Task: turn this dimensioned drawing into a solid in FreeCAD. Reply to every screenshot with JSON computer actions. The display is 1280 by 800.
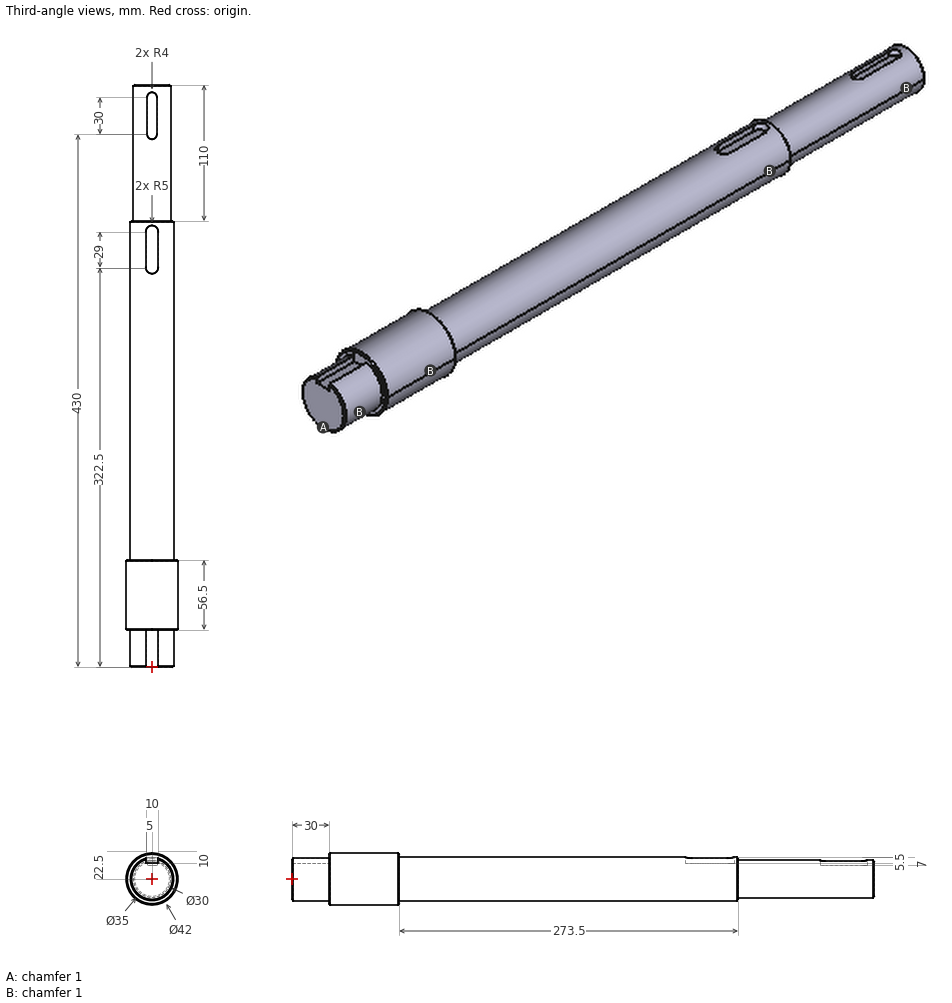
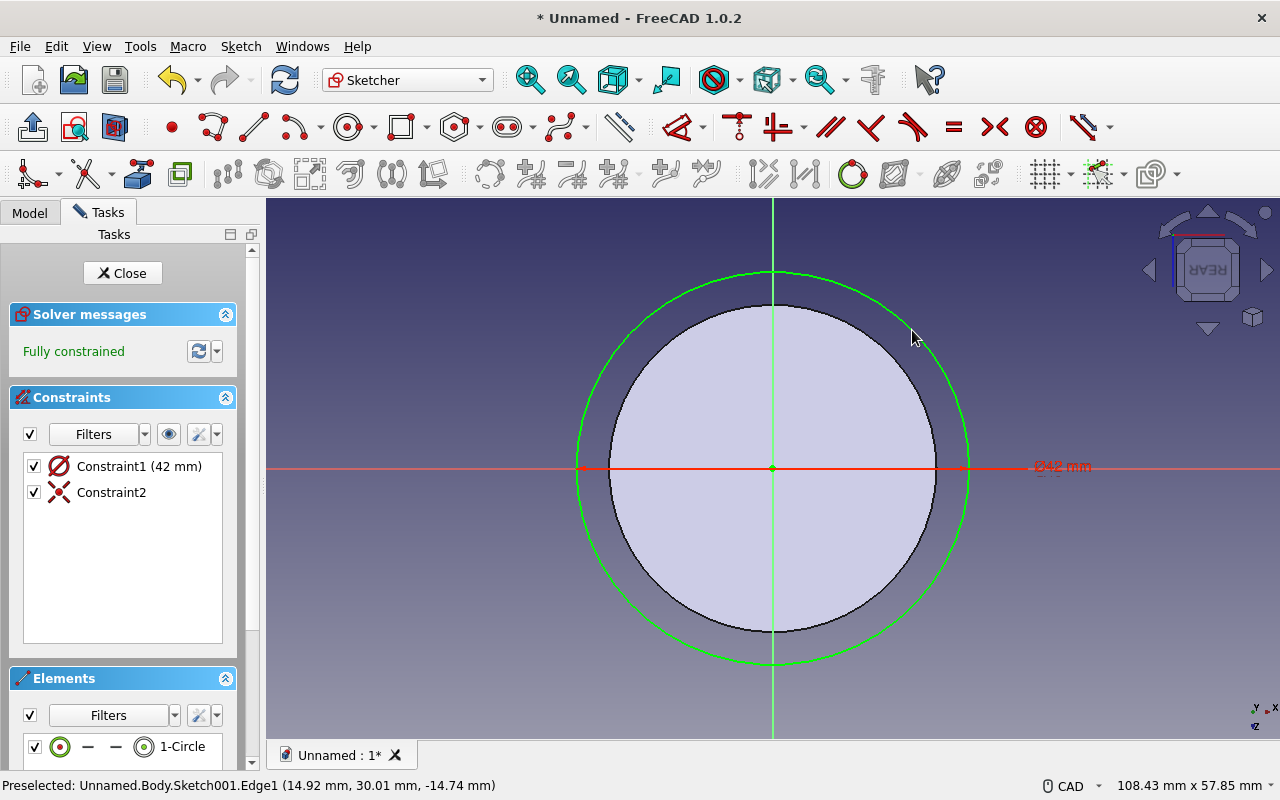
{"action": "left_click", "coordinate": [123, 273]}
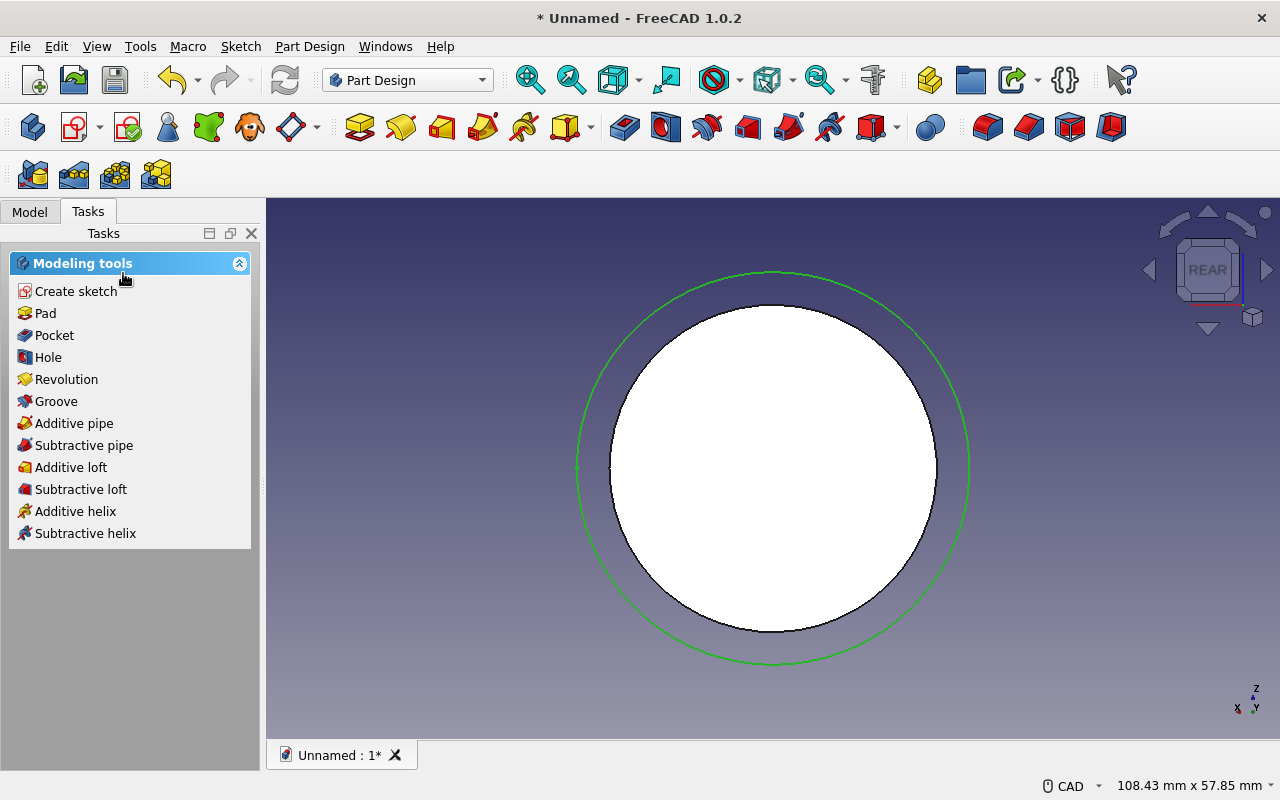
{"action": "left_click", "coordinate": [360, 128]}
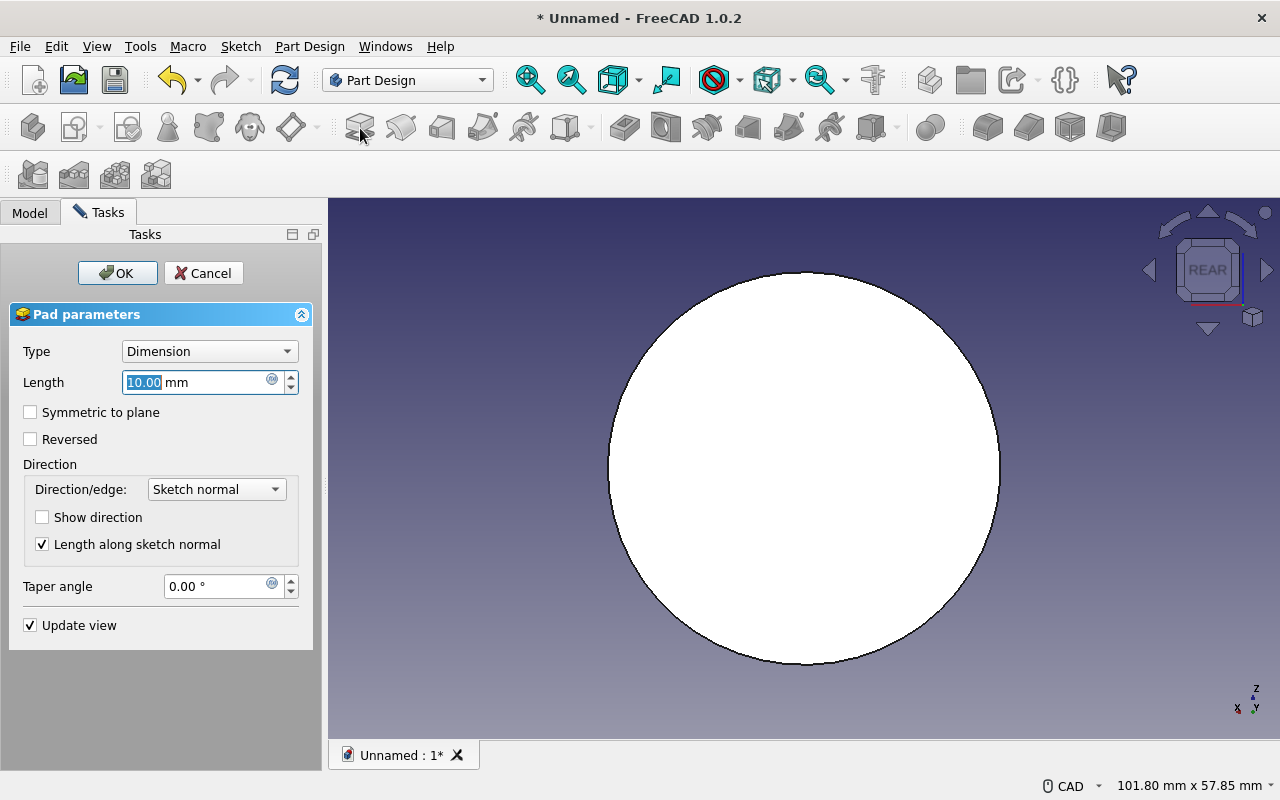
{"action": "type", "text": "56.5"}
{"action": "key", "text": "Tab"}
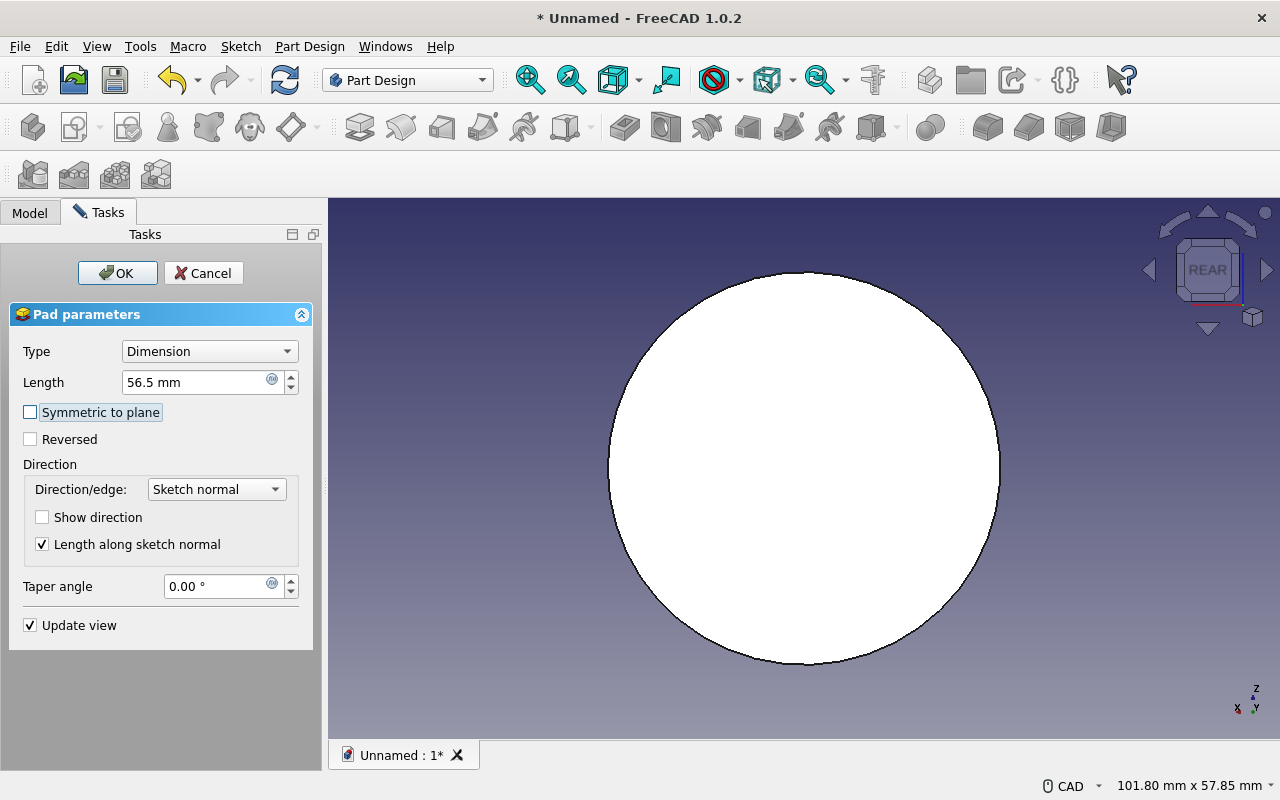
{"action": "left_click", "coordinate": [118, 273]}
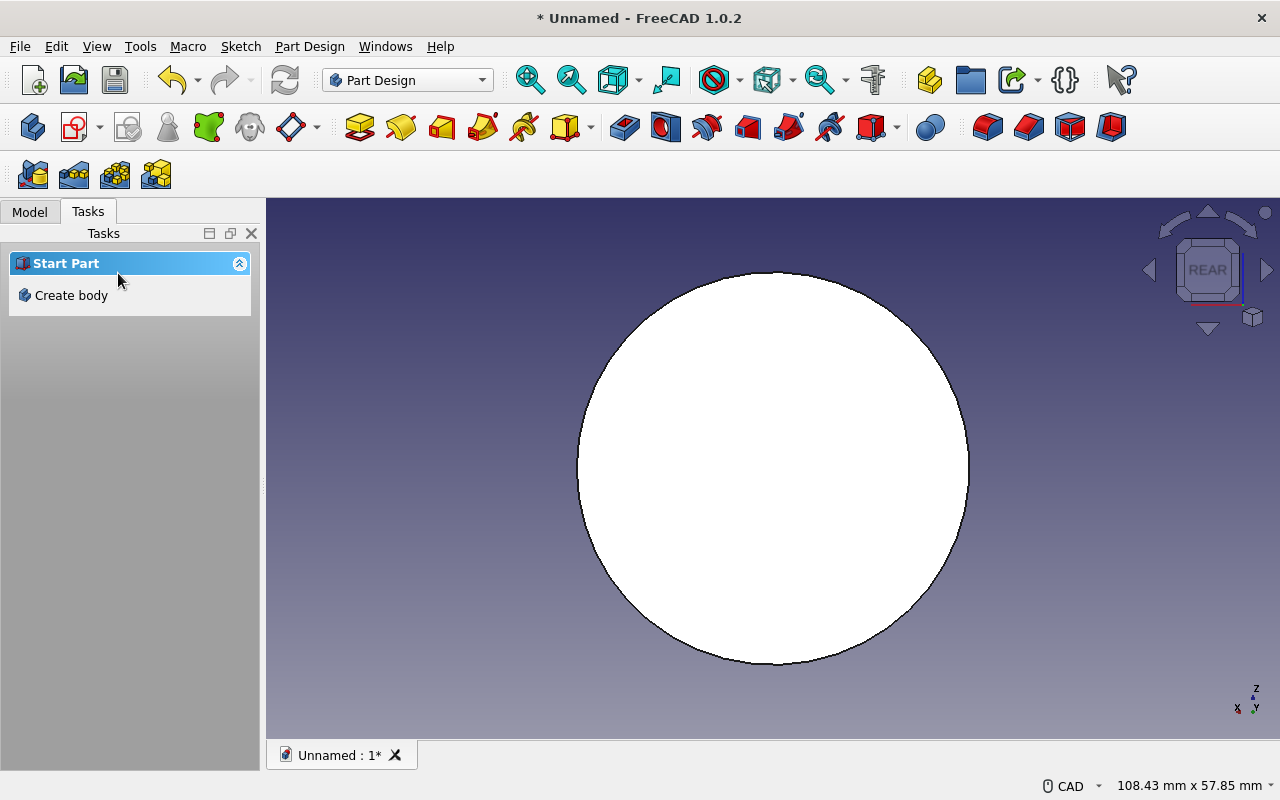
{"action": "left_click", "coordinate": [773, 468]}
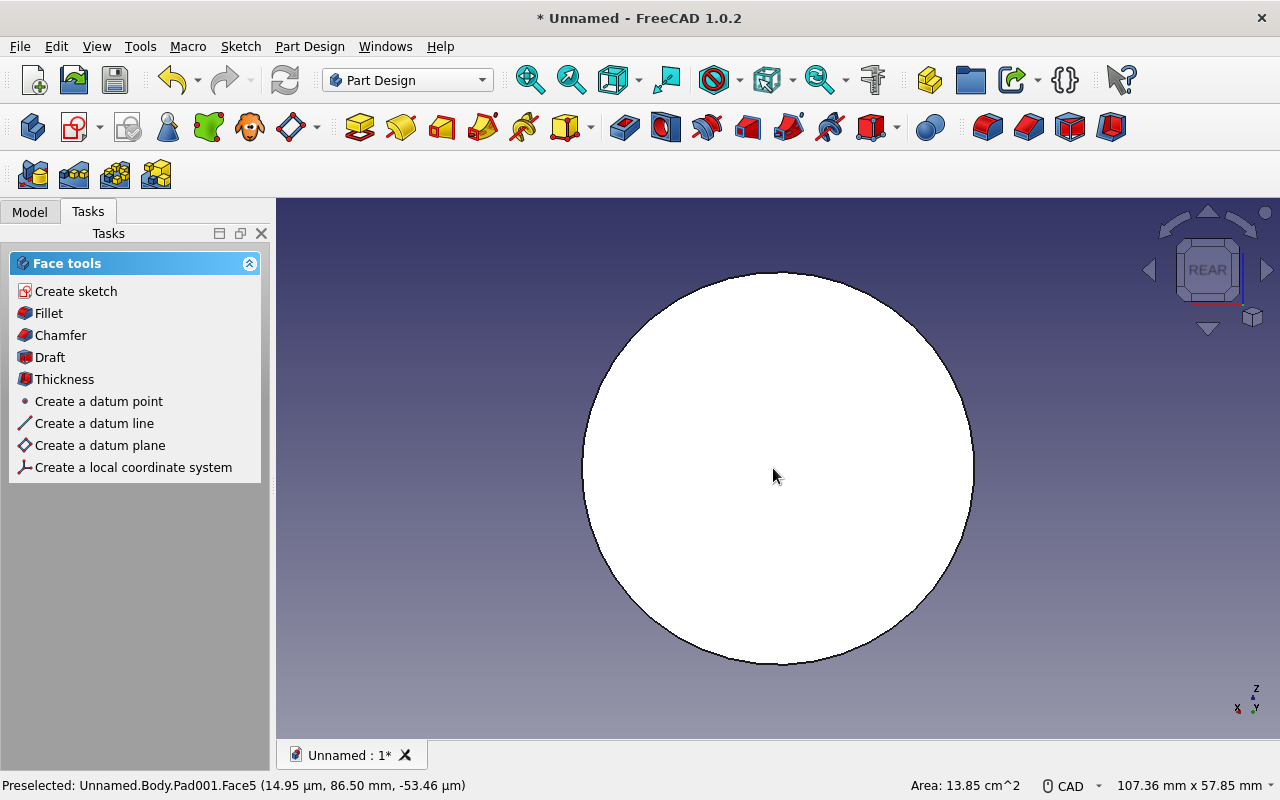
{"action": "left_click", "coordinate": [74, 128]}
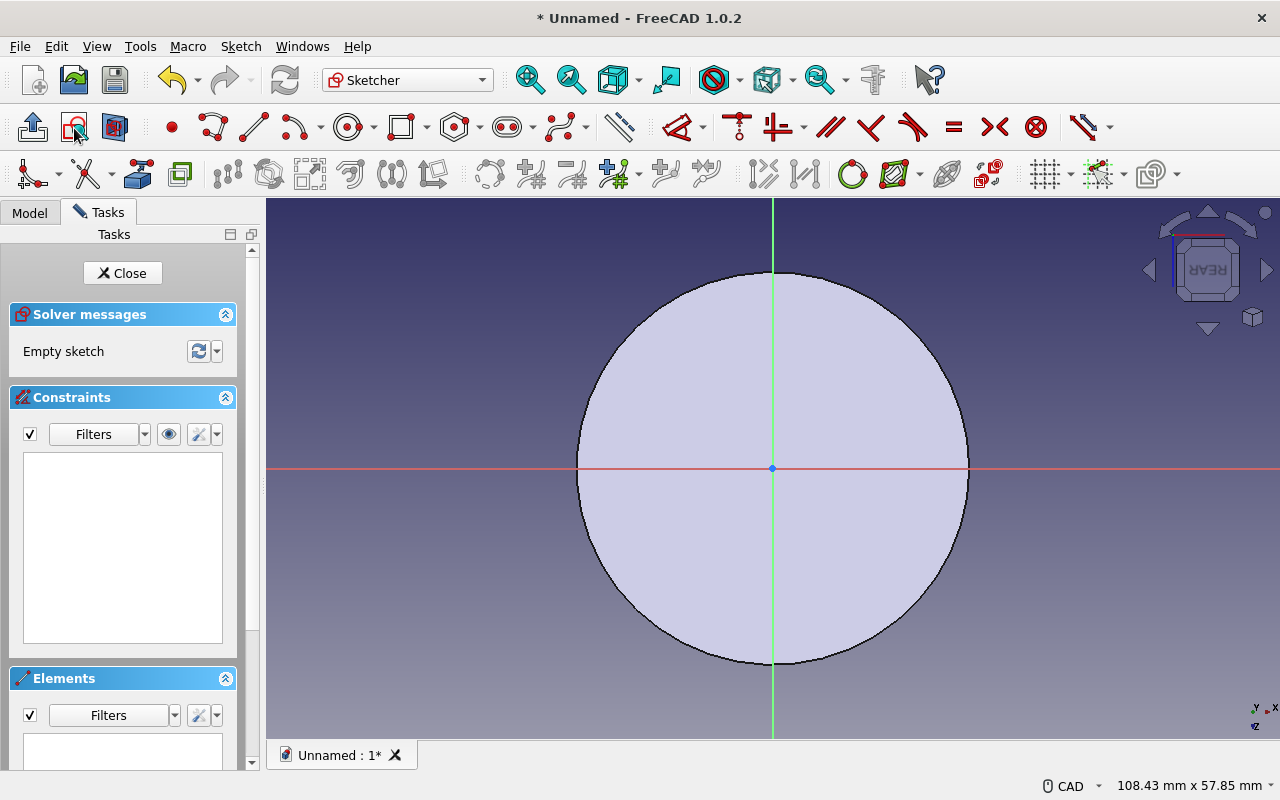
{"action": "left_click", "coordinate": [348, 128]}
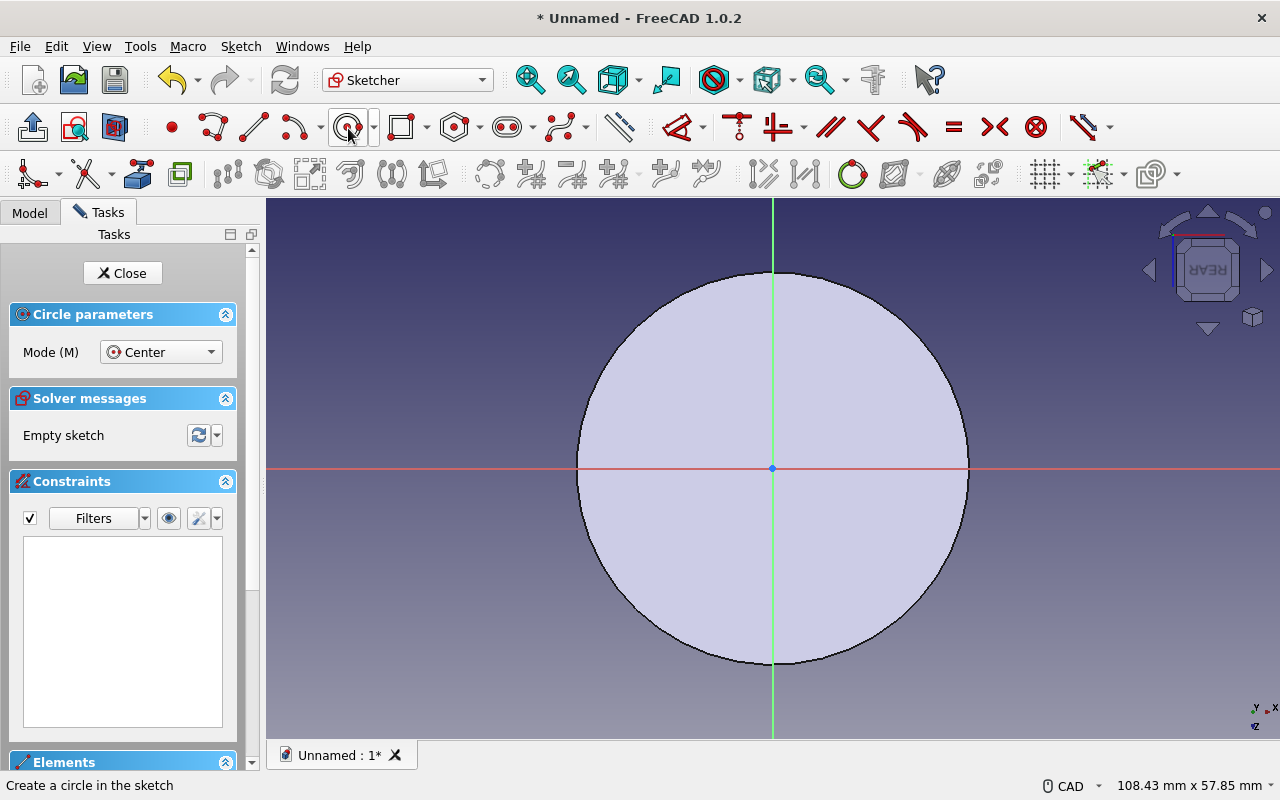
{"action": "left_click", "coordinate": [773, 468]}
{"action": "mouse_move", "coordinate": [889, 353]}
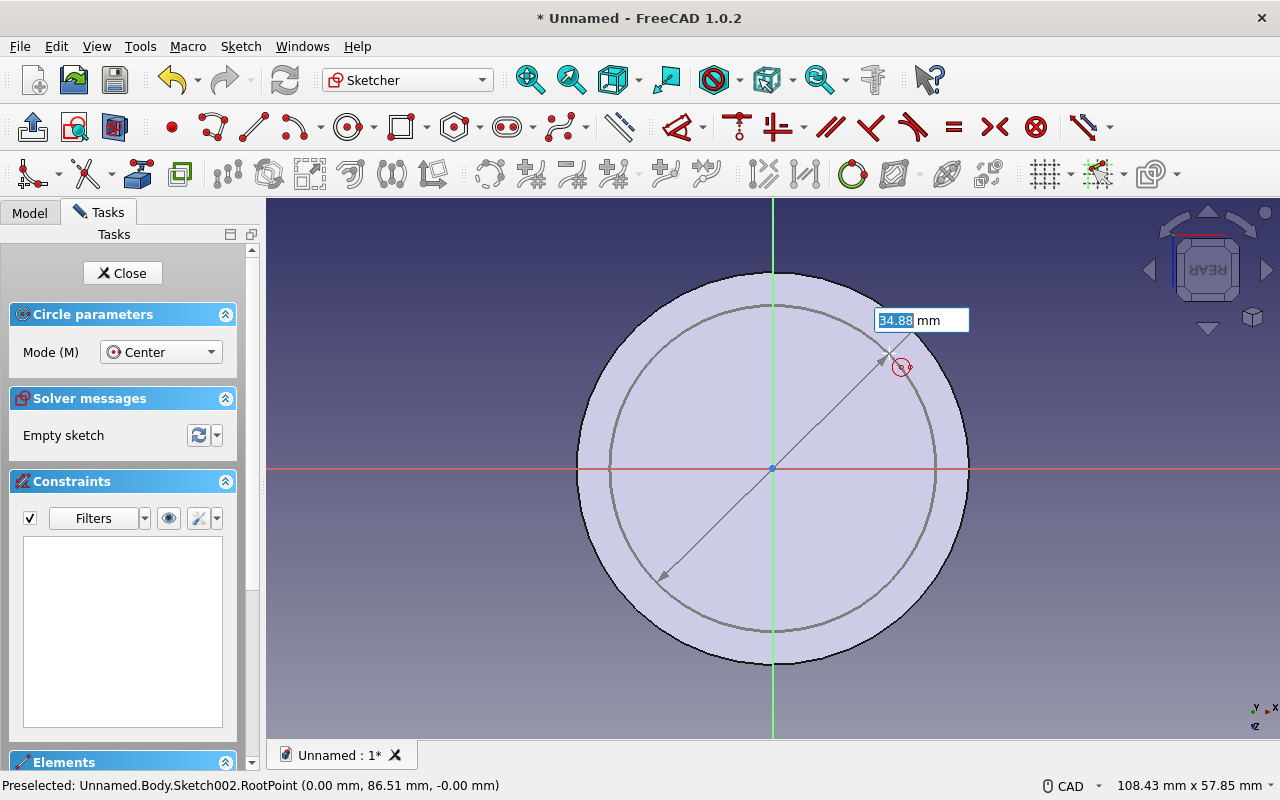
{"action": "type", "text": "35"}
{"action": "key", "text": "Return"}
{"action": "key", "text": "Escape"}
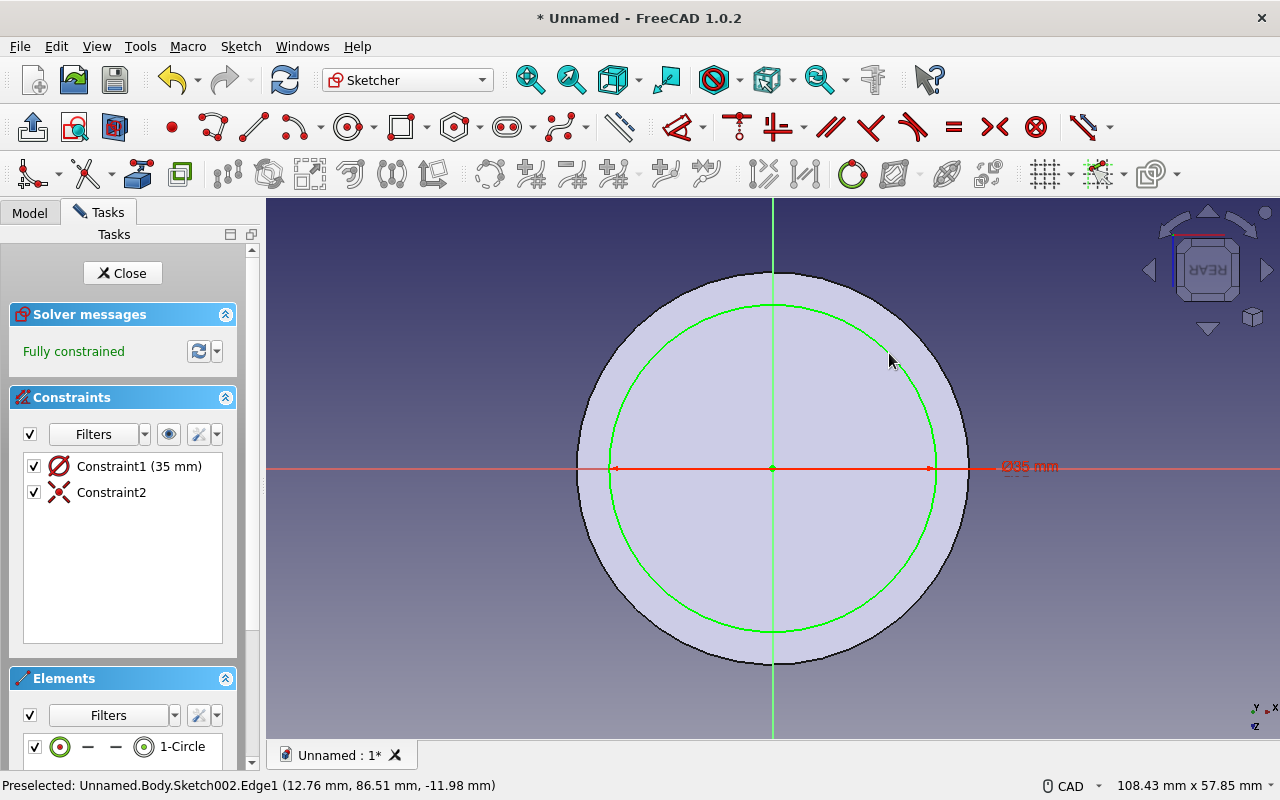
{"action": "left_click", "coordinate": [123, 273]}